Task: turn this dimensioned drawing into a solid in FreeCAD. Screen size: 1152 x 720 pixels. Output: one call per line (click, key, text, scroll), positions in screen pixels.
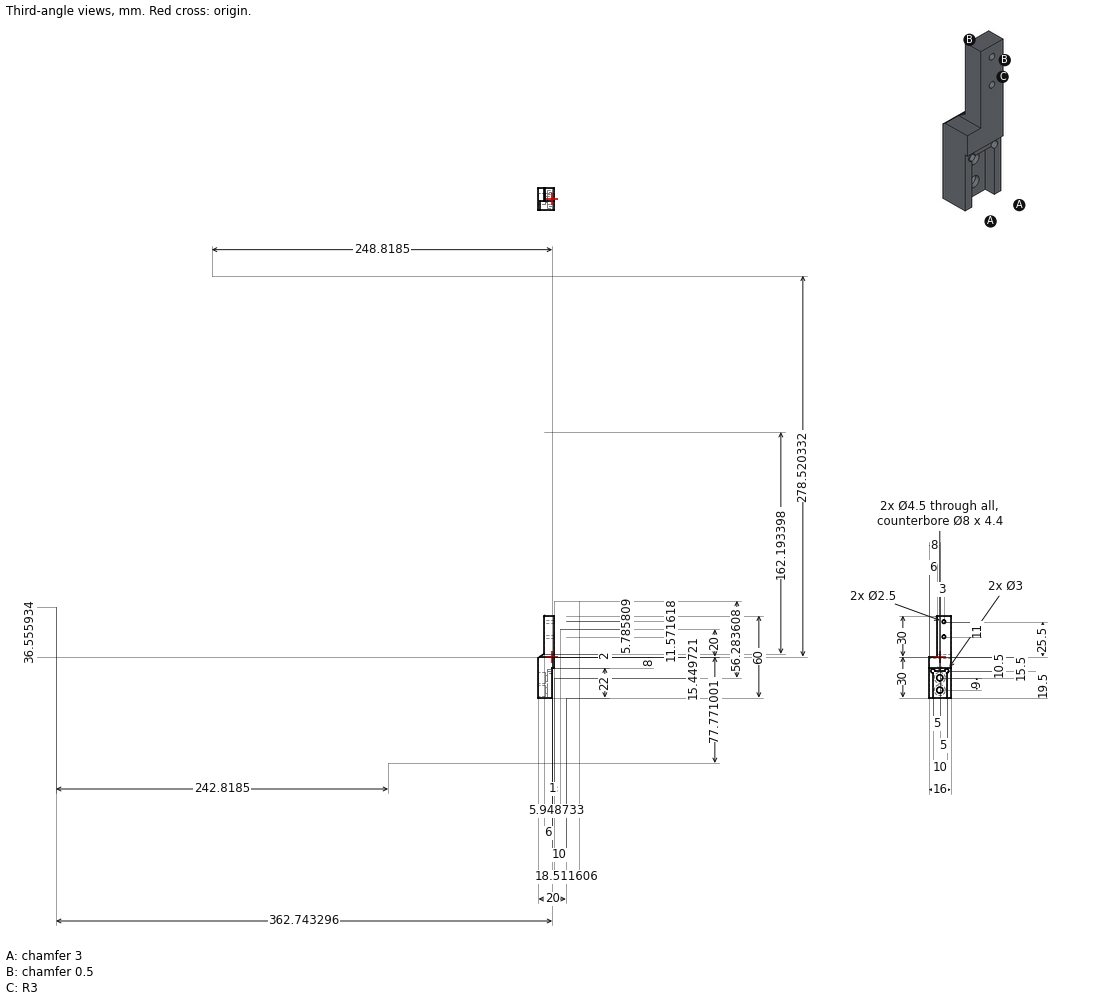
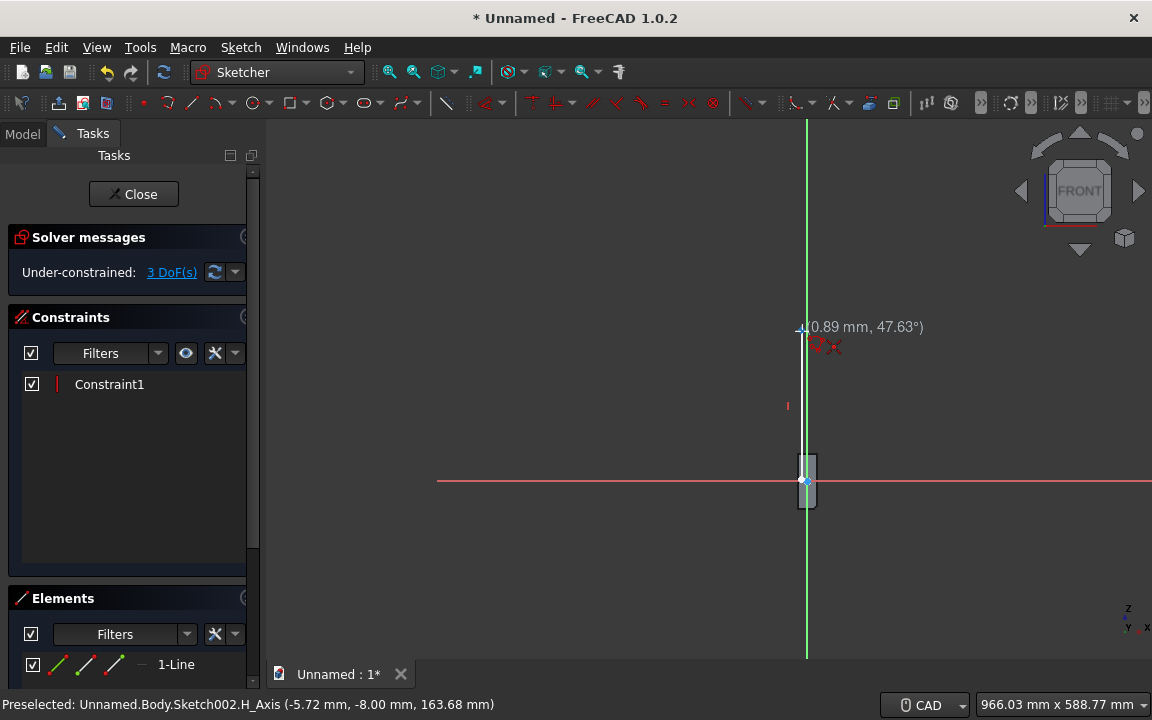
click(579, 226)
click(475, 448)
click(697, 553)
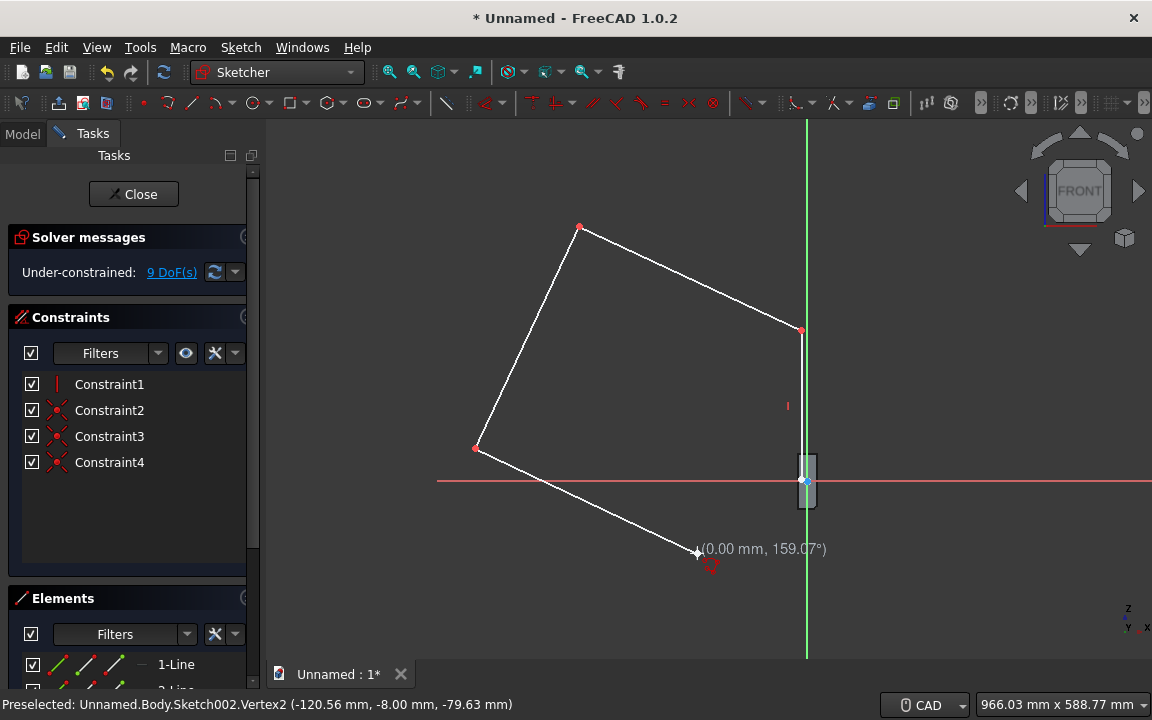
scroll(802, 480, up, 11)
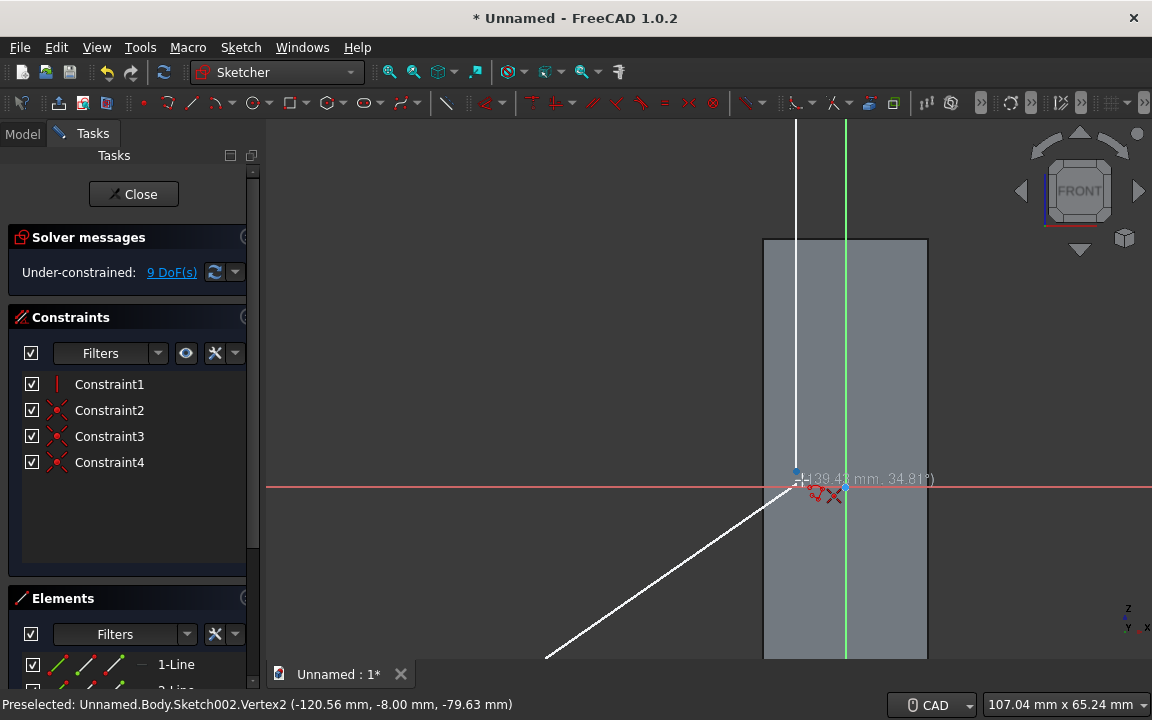
click(796, 472)
key(Escape)
key(Escape)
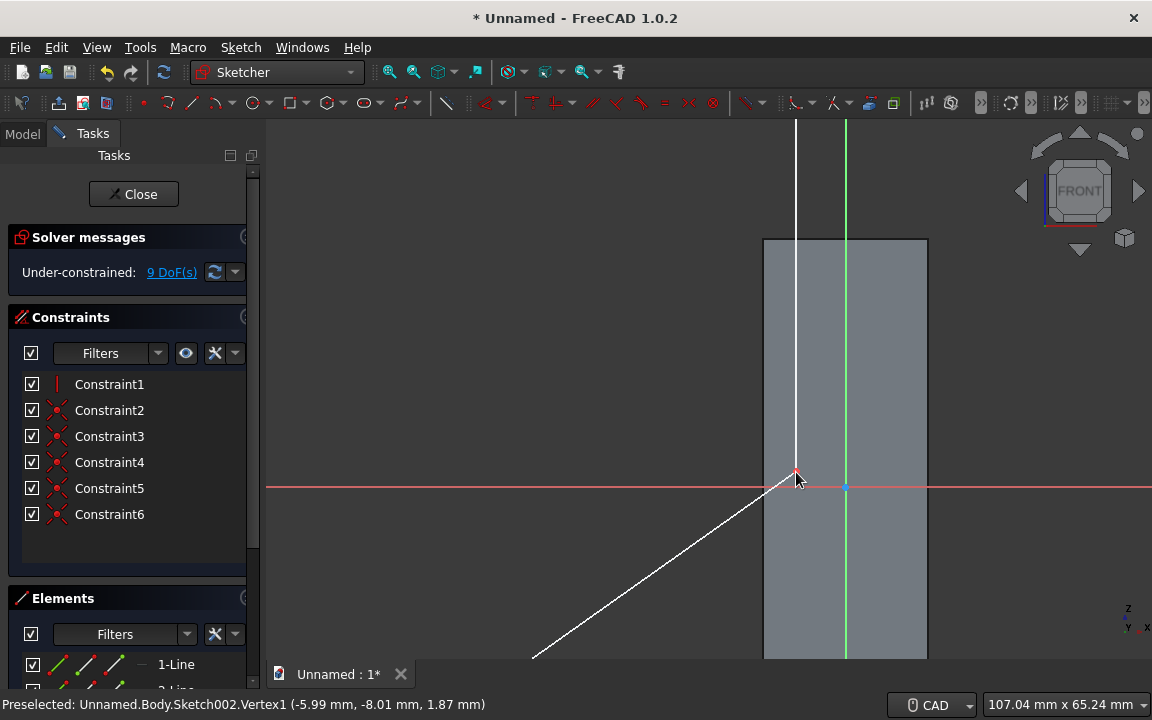
key(d)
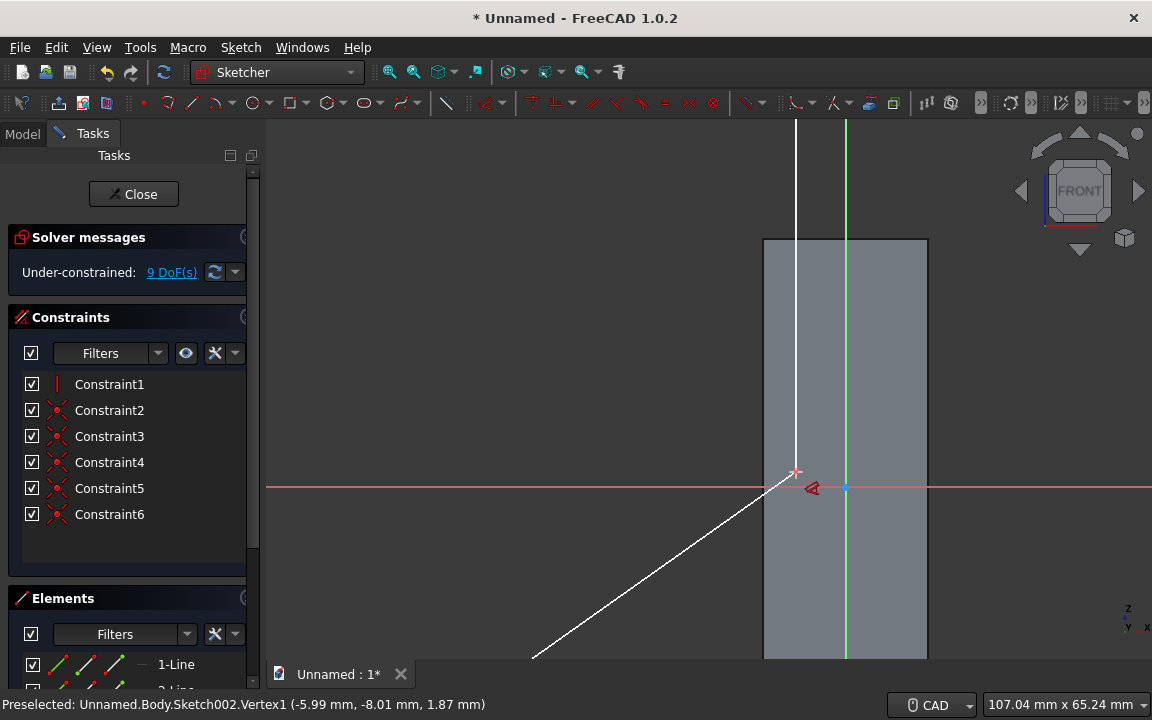
click(796, 472)
click(821, 521)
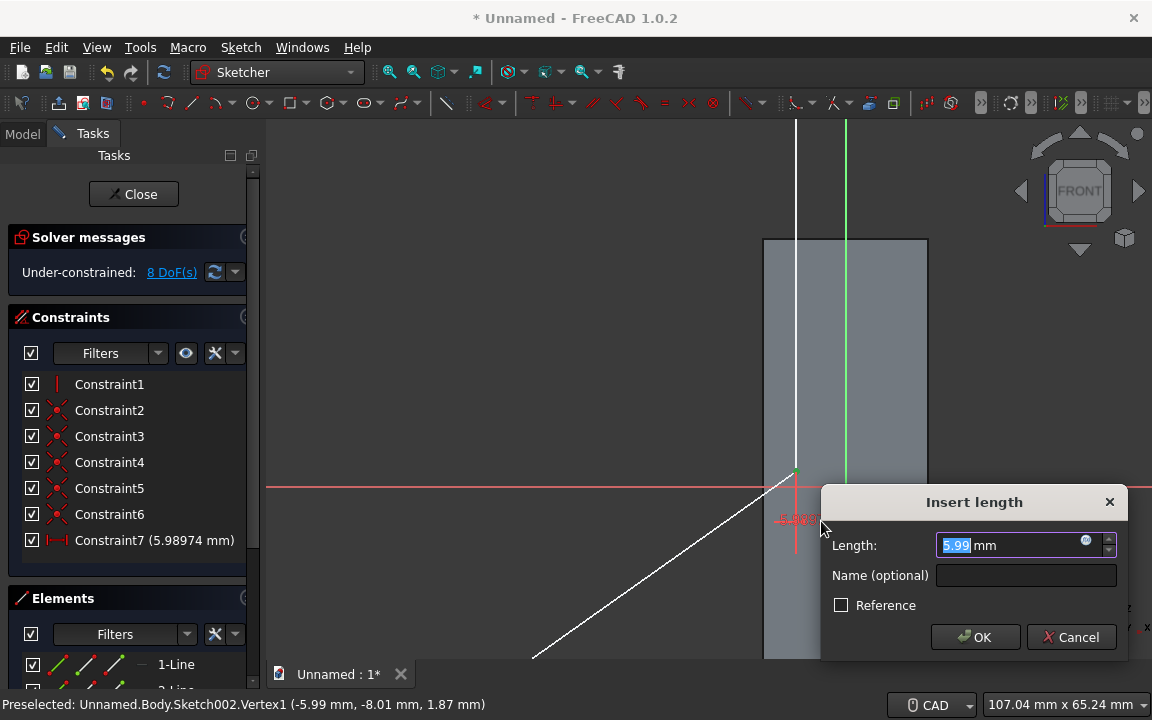
text(6)
key(Return)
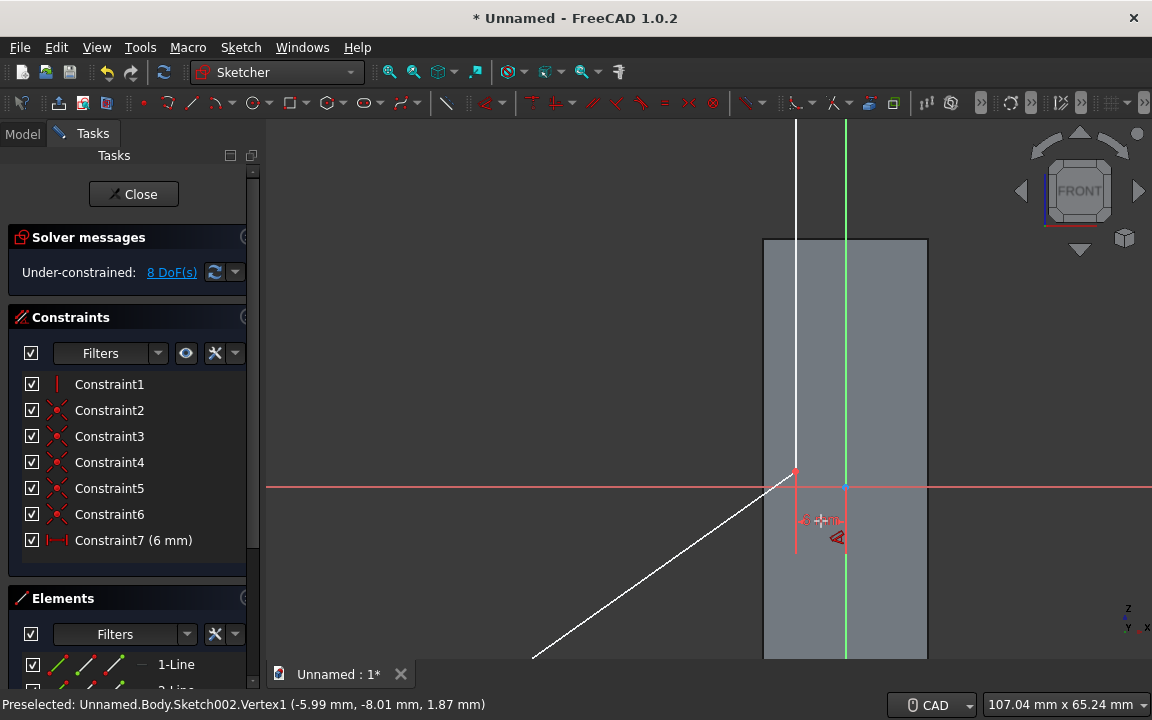
scroll(796, 472, up, 5)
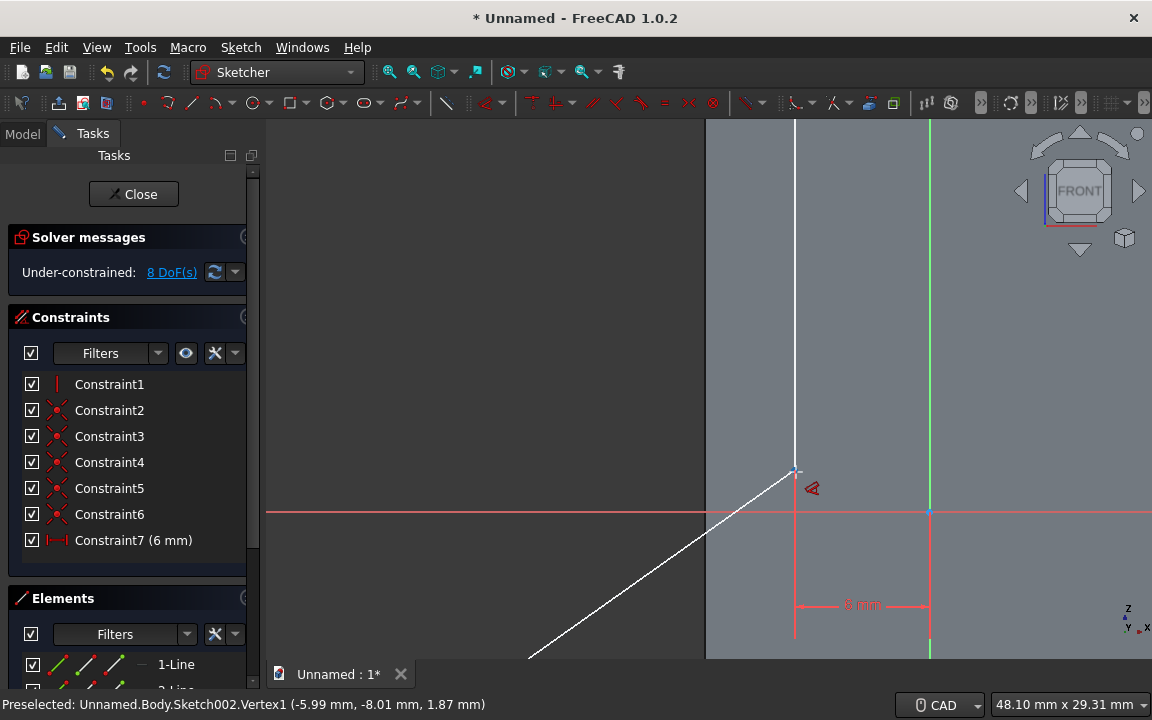
click(795, 470)
click(964, 491)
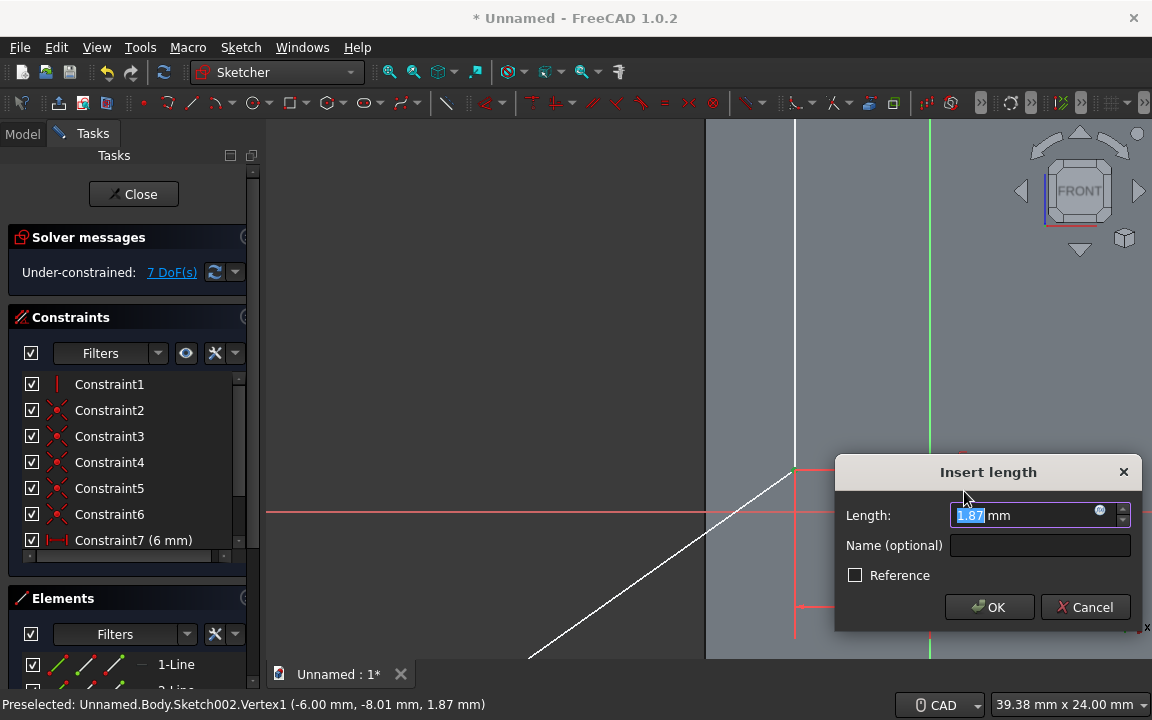
text(2)
key(Return)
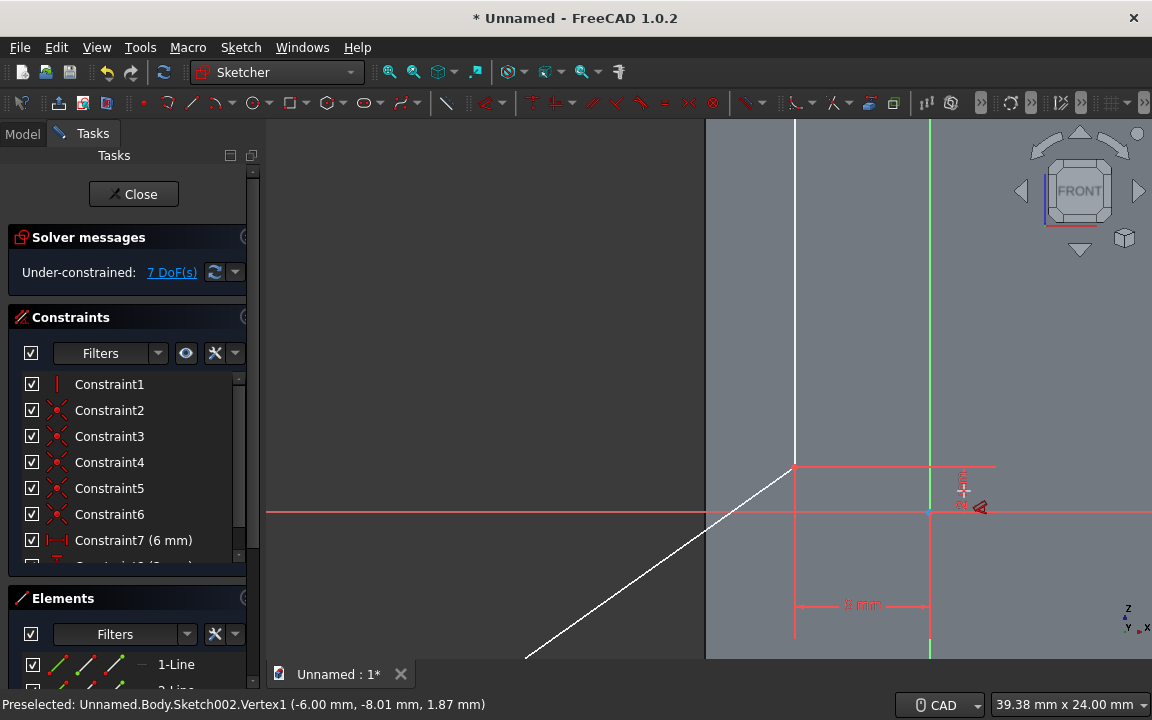
scroll(839, 501, down, 15)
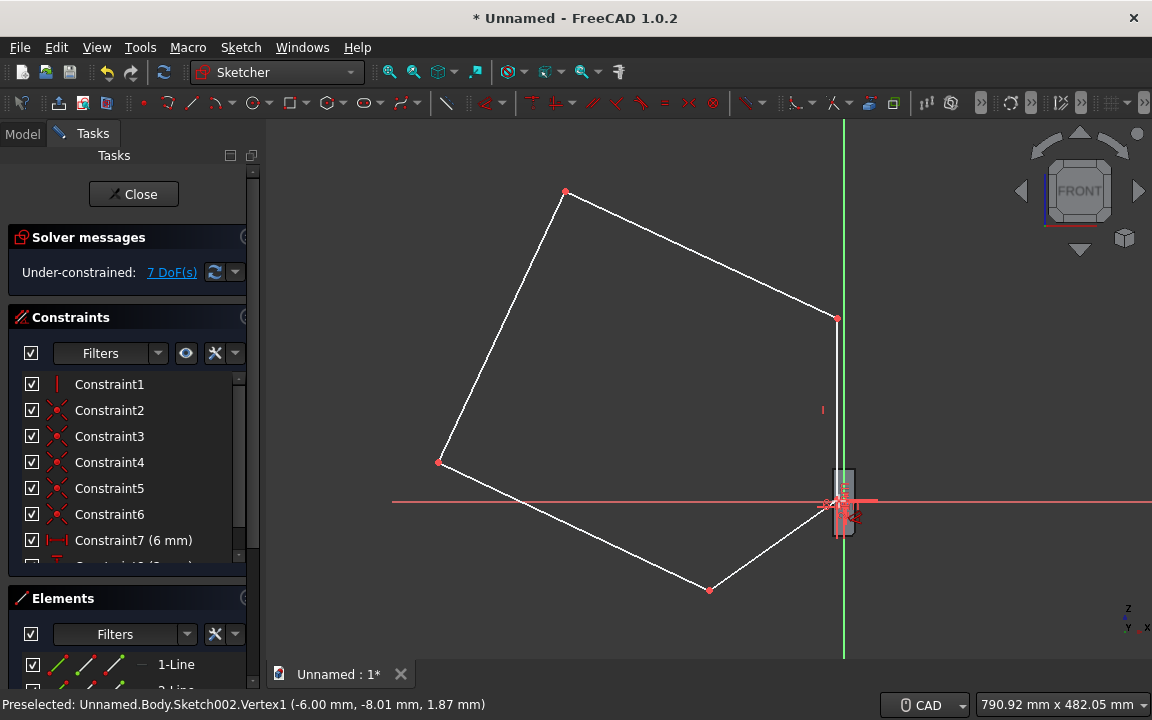
click(565, 192)
click(705, 158)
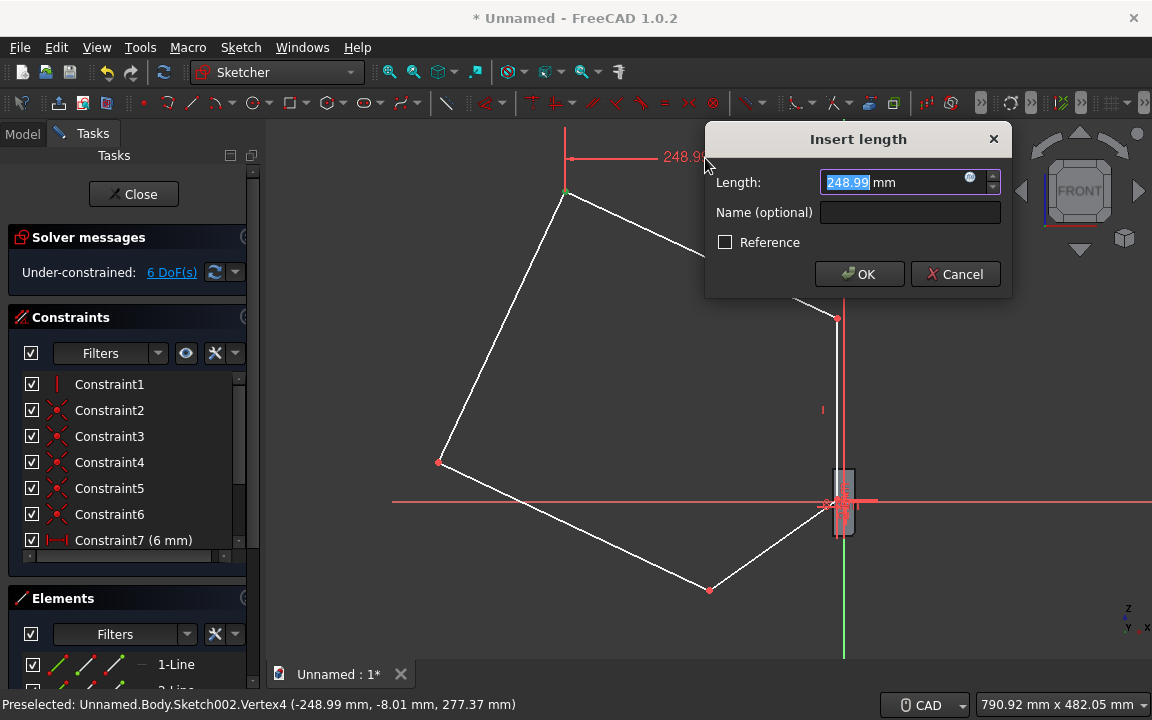
text(248.8185)
key(Return)